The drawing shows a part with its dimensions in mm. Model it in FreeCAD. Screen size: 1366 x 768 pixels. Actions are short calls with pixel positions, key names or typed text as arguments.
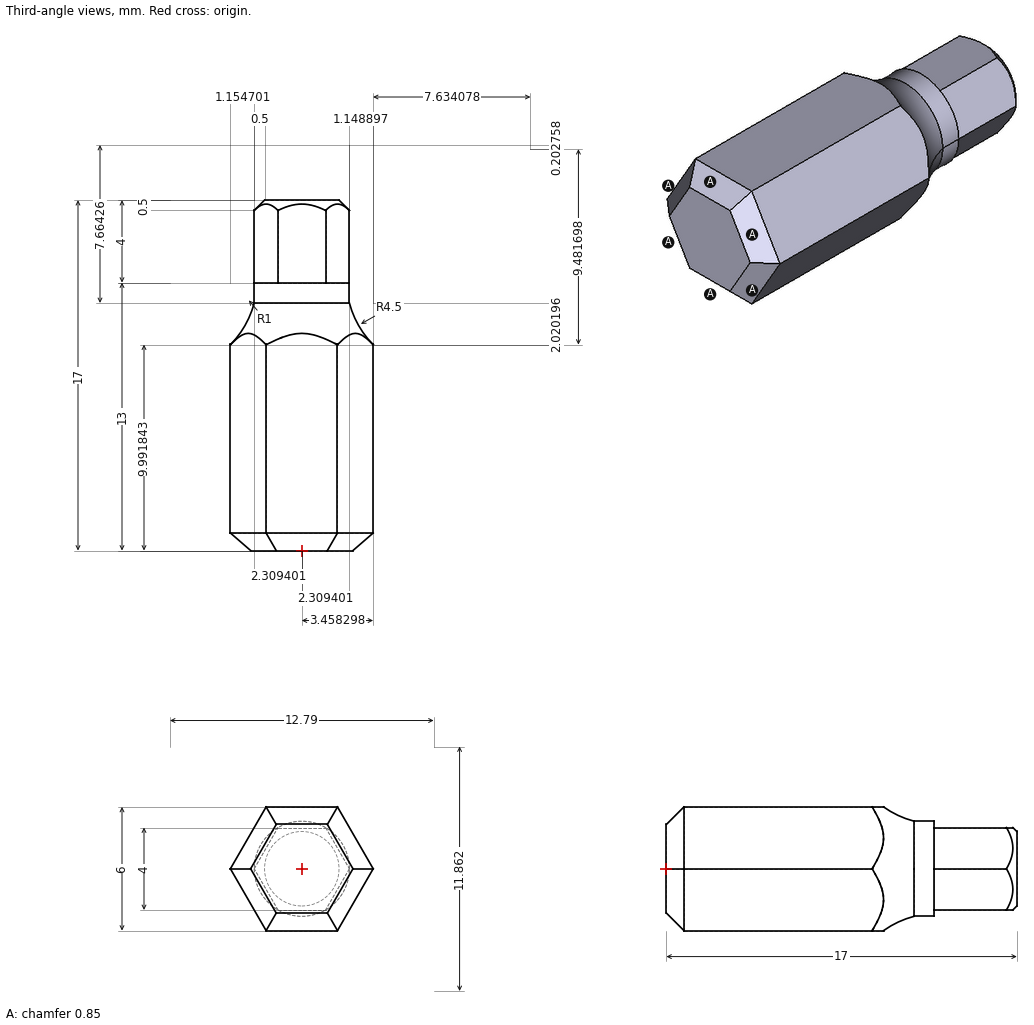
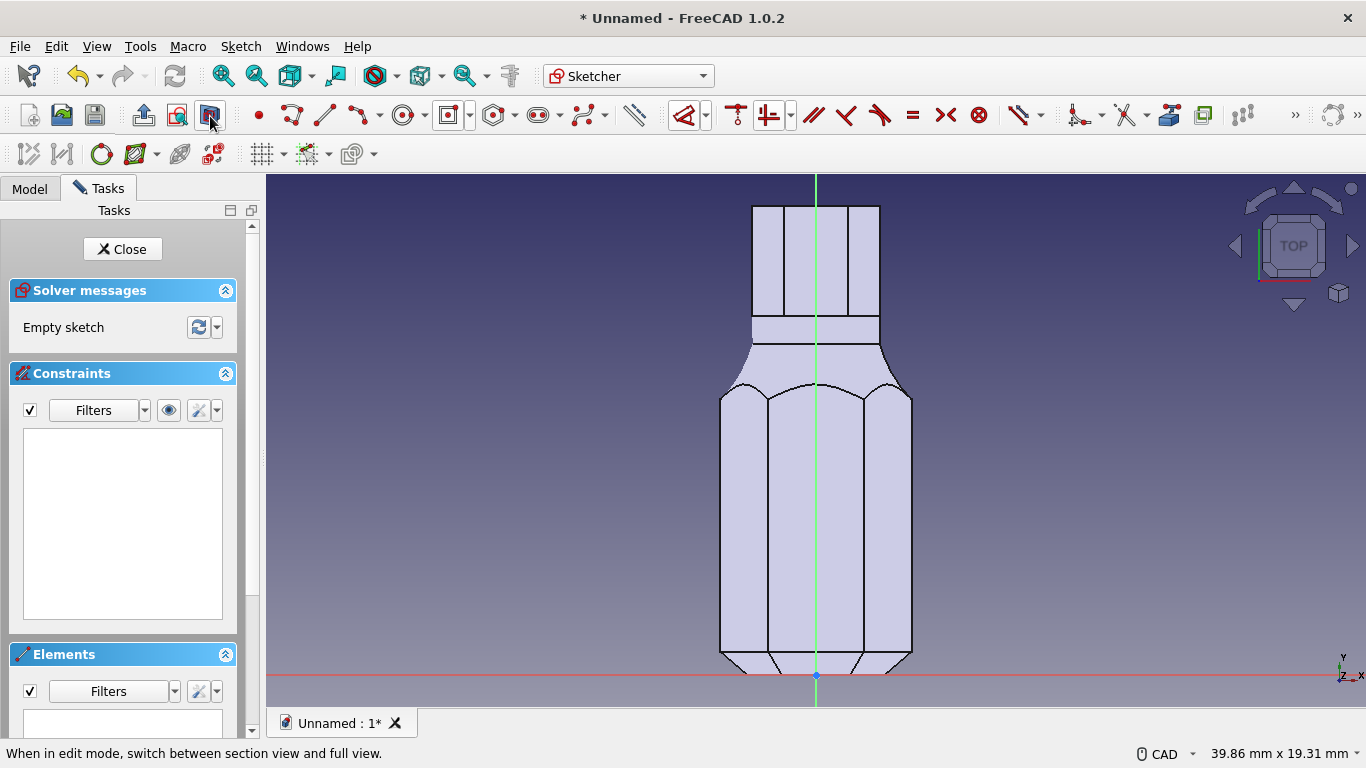
scroll(760, 202, up, 15)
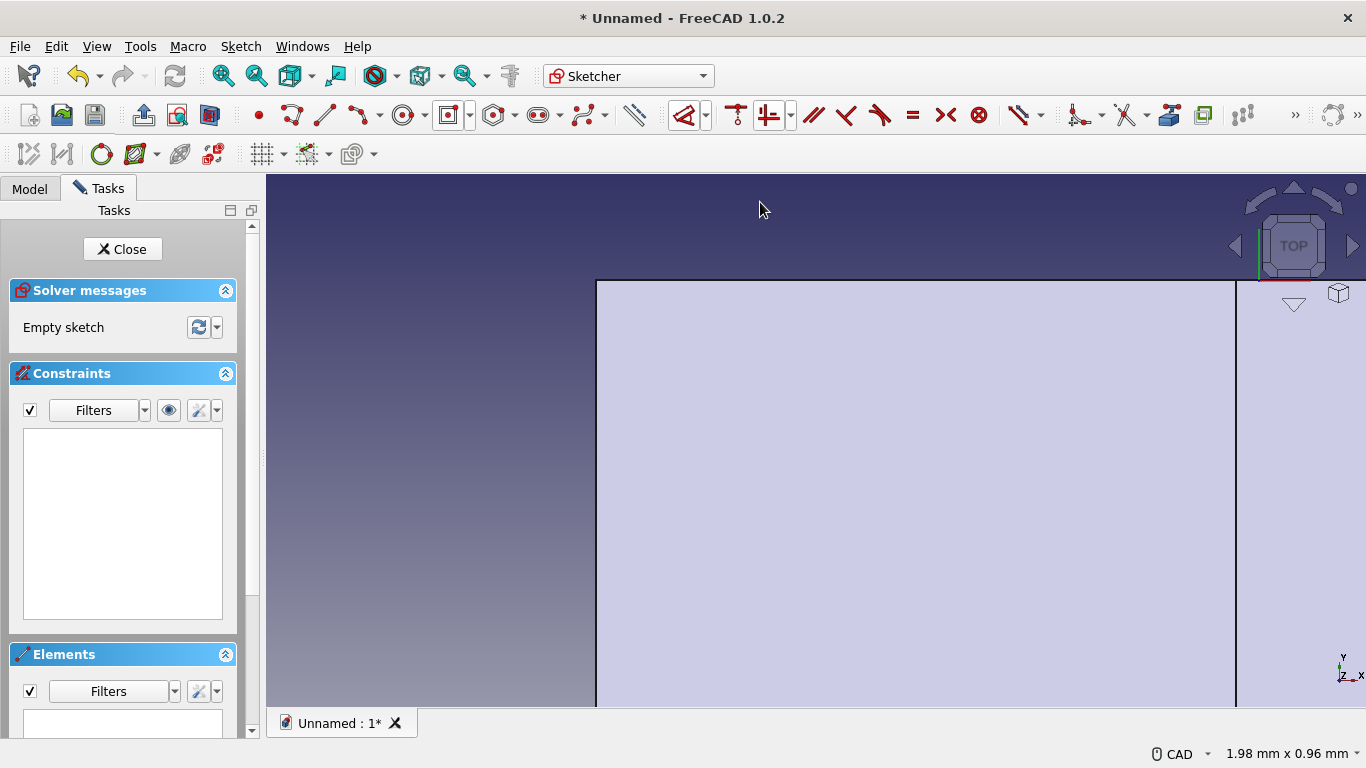
click(292, 116)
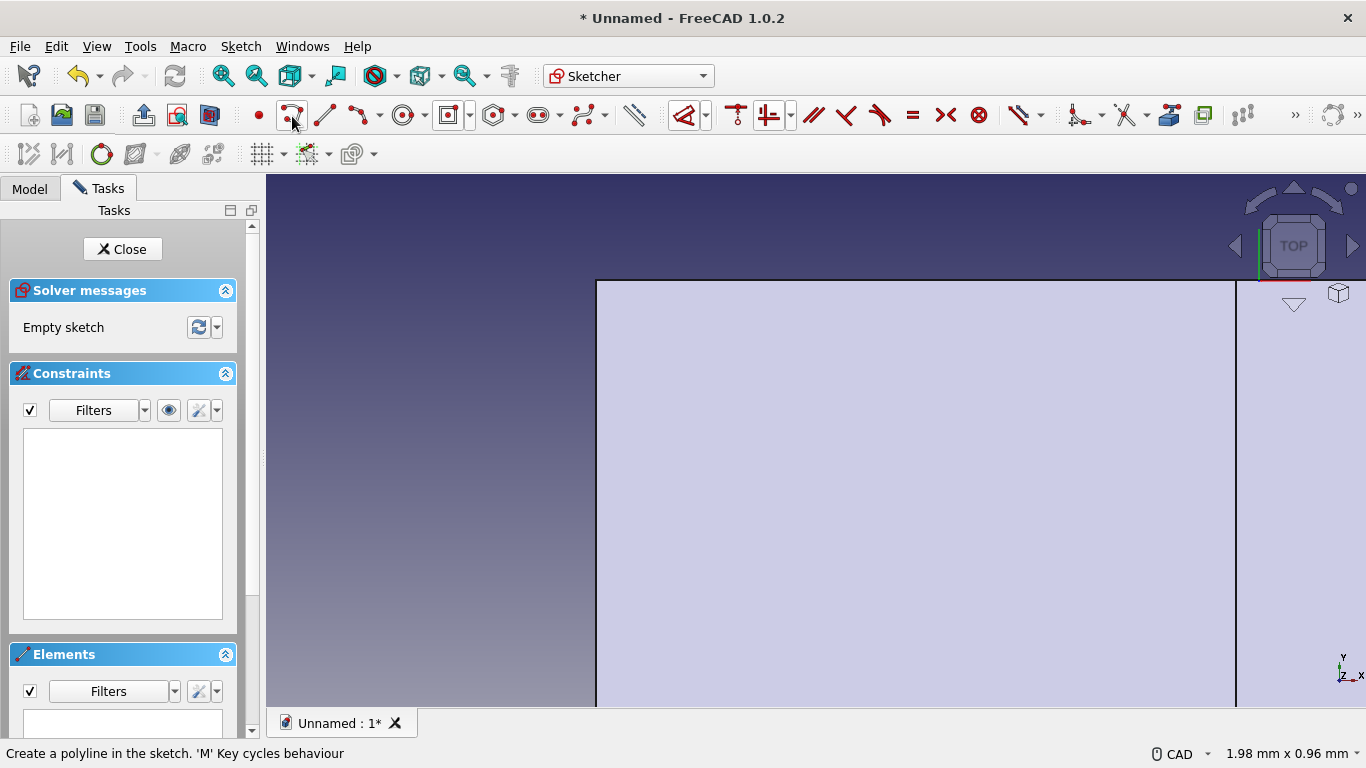
click(596, 557)
click(873, 280)
click(596, 280)
click(596, 558)
key(Escape)
key(Escape)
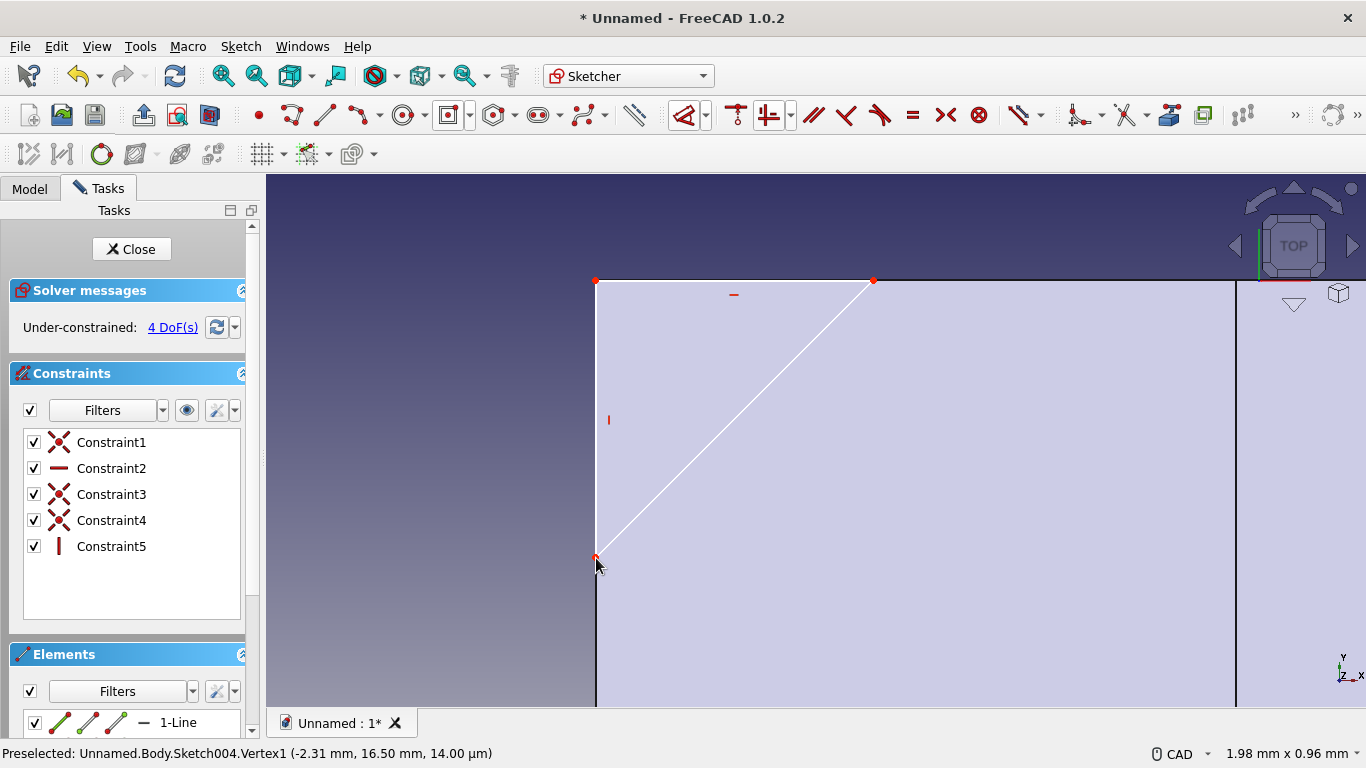
click(790, 281)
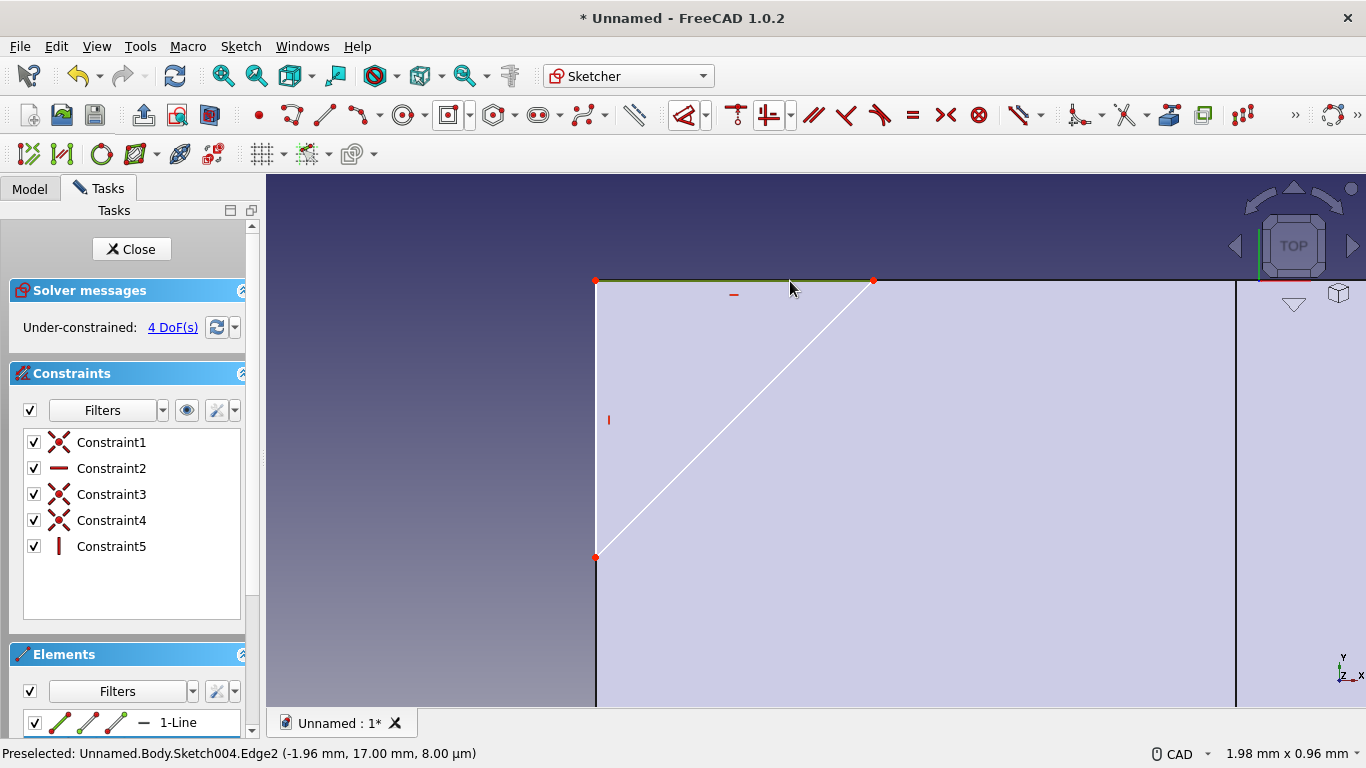
click(706, 116)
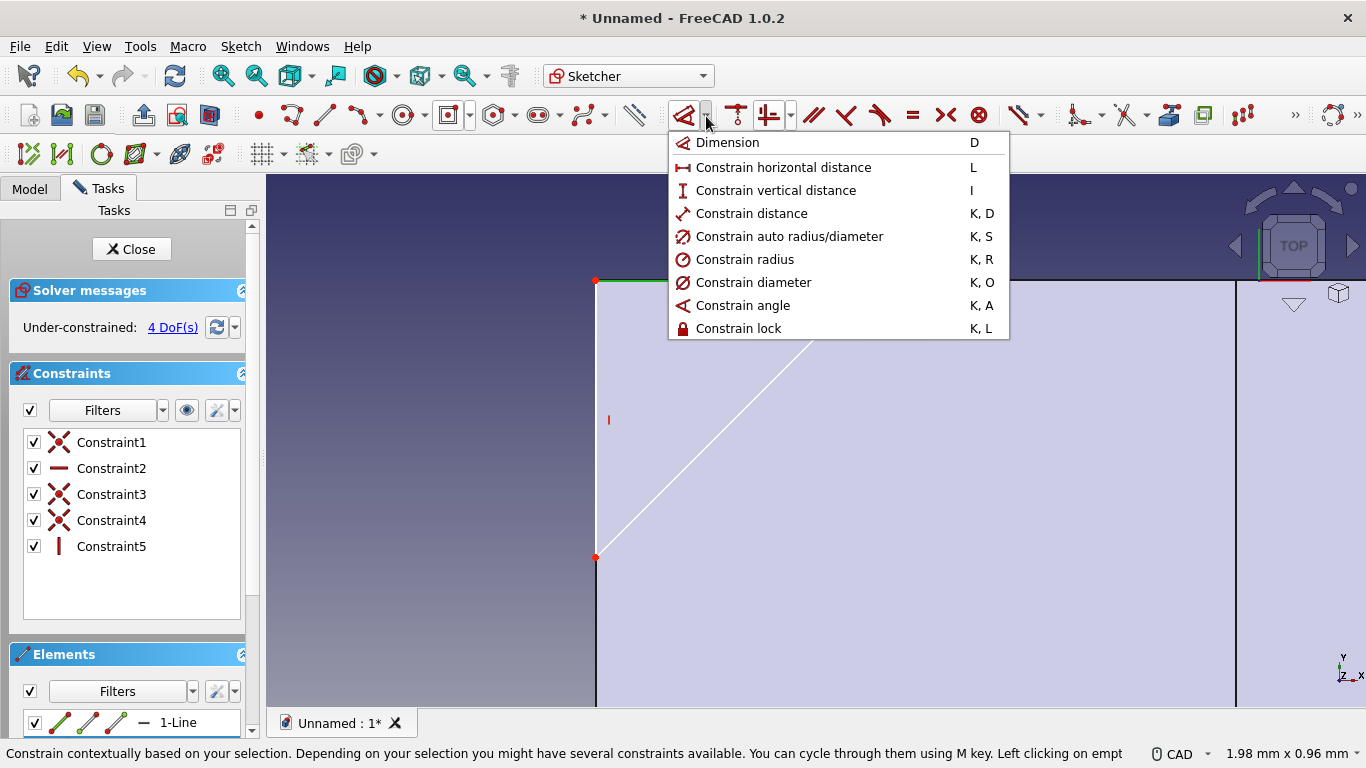
click(839, 168)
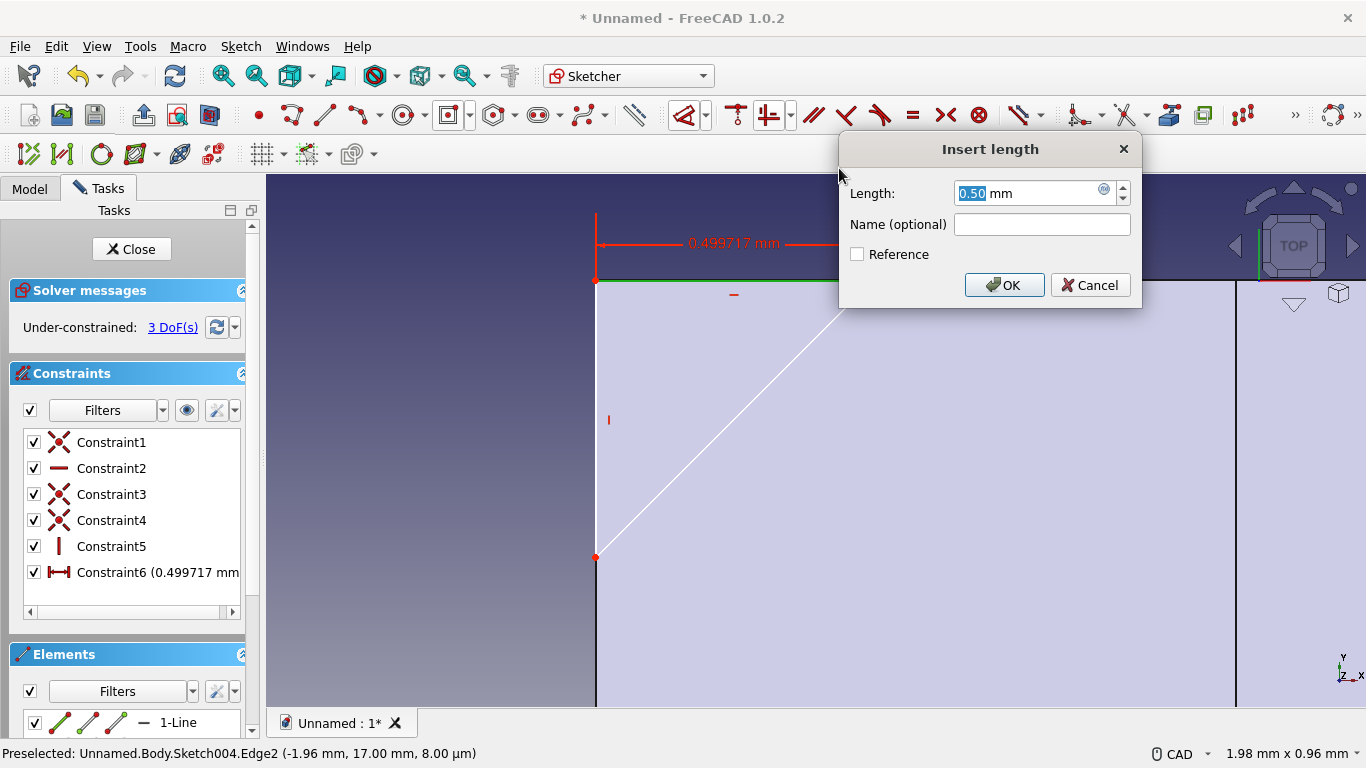
text(0.5)
key(Return)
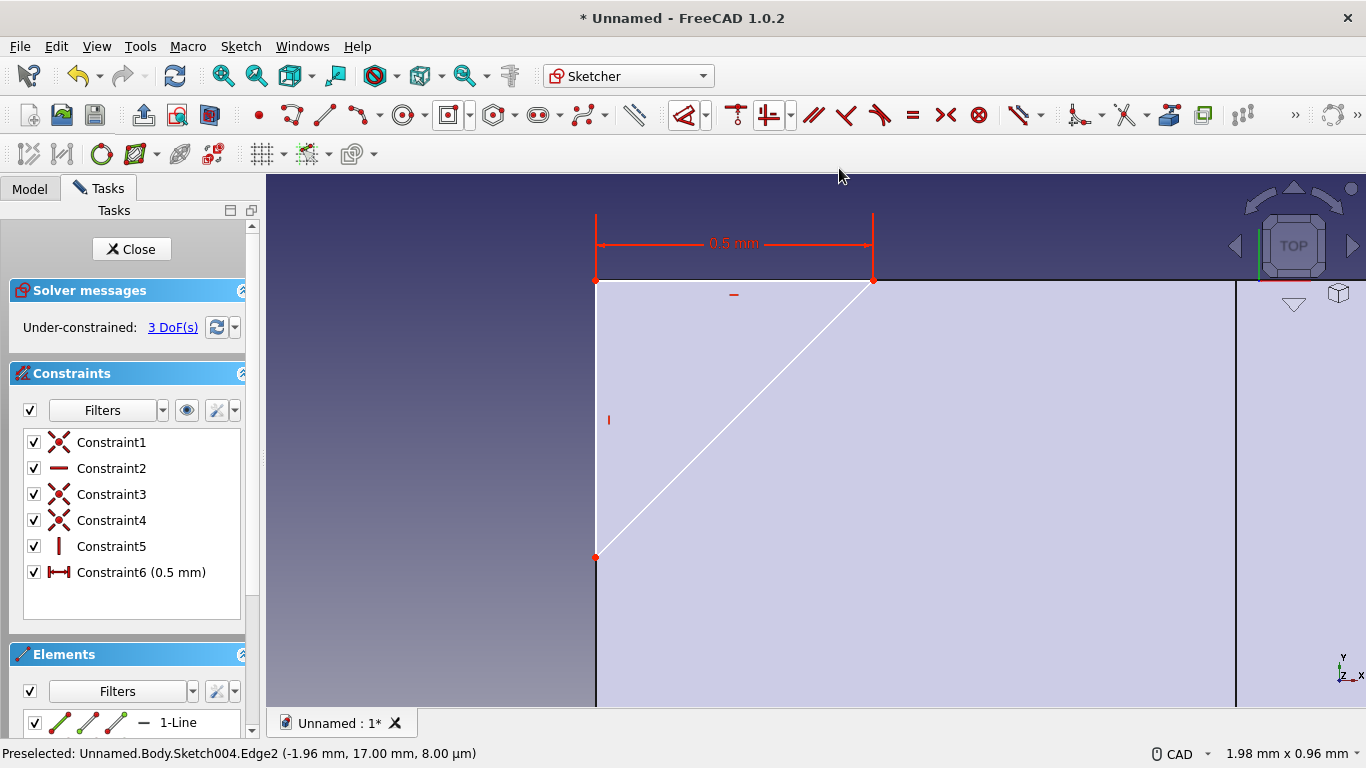
click(596, 364)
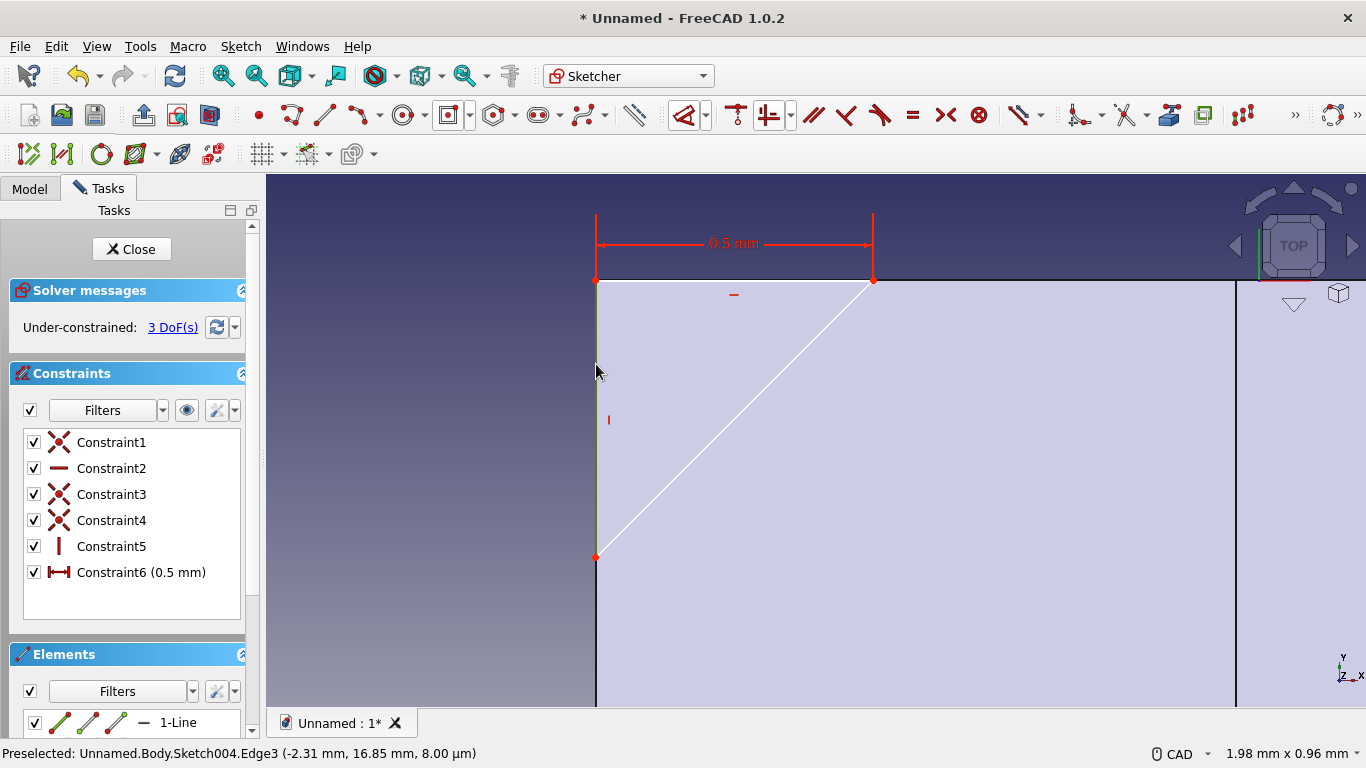
click(706, 116)